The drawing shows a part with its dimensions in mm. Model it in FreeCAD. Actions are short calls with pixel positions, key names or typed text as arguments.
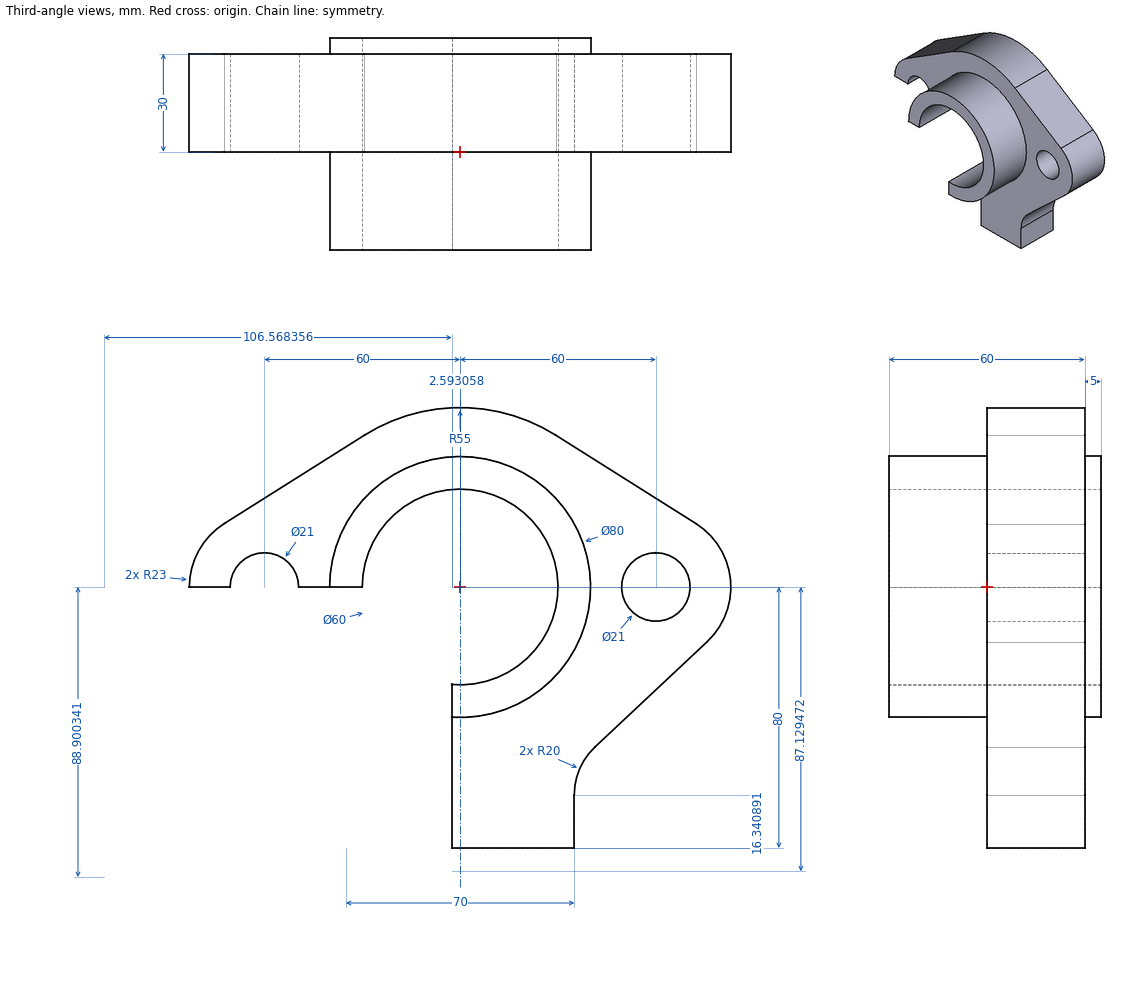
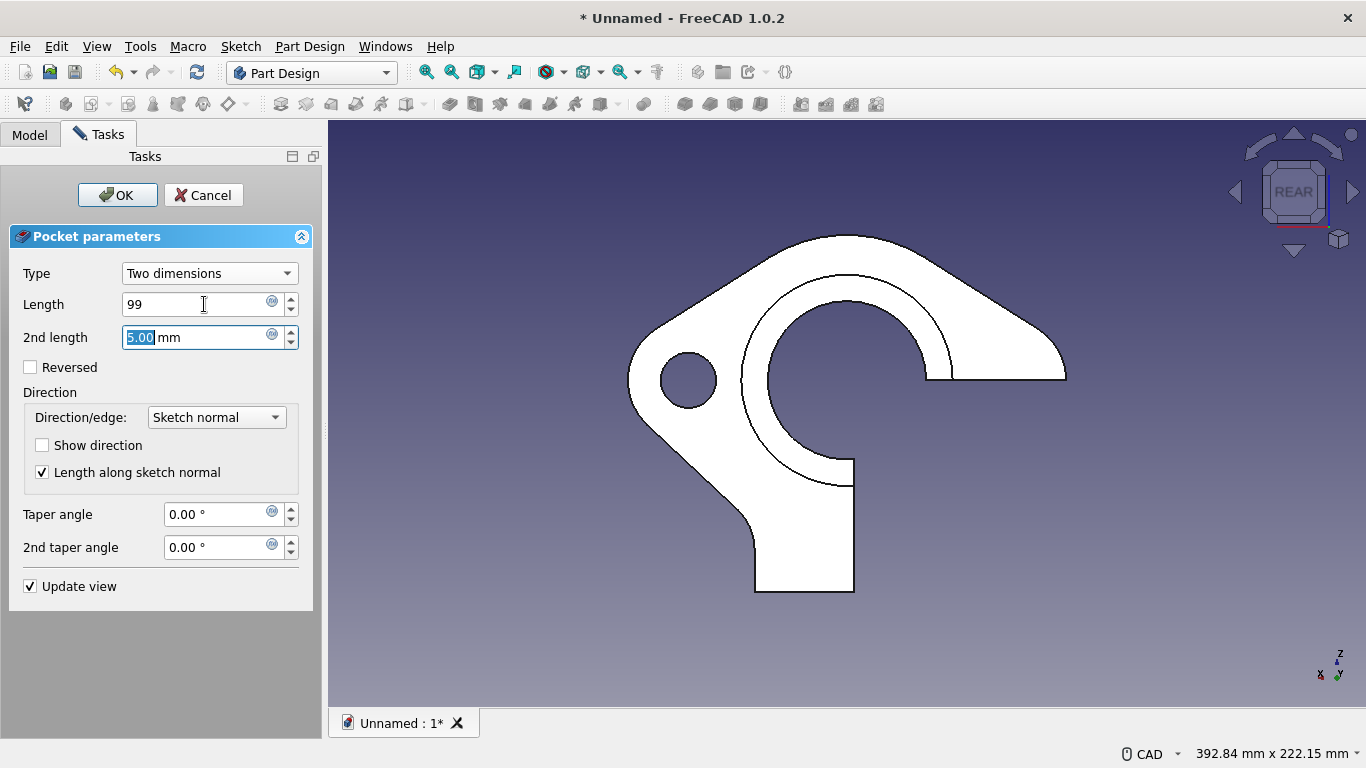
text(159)
key(Tab)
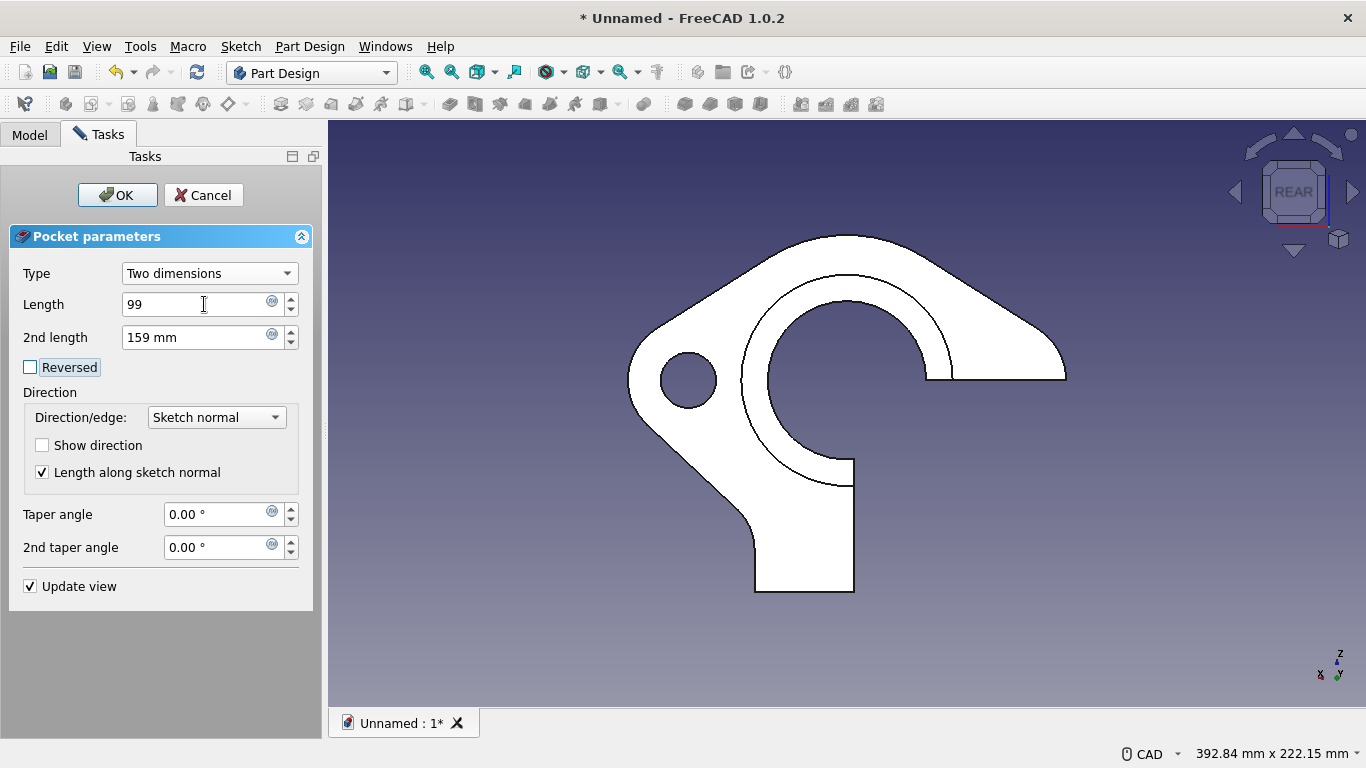
click(31, 367)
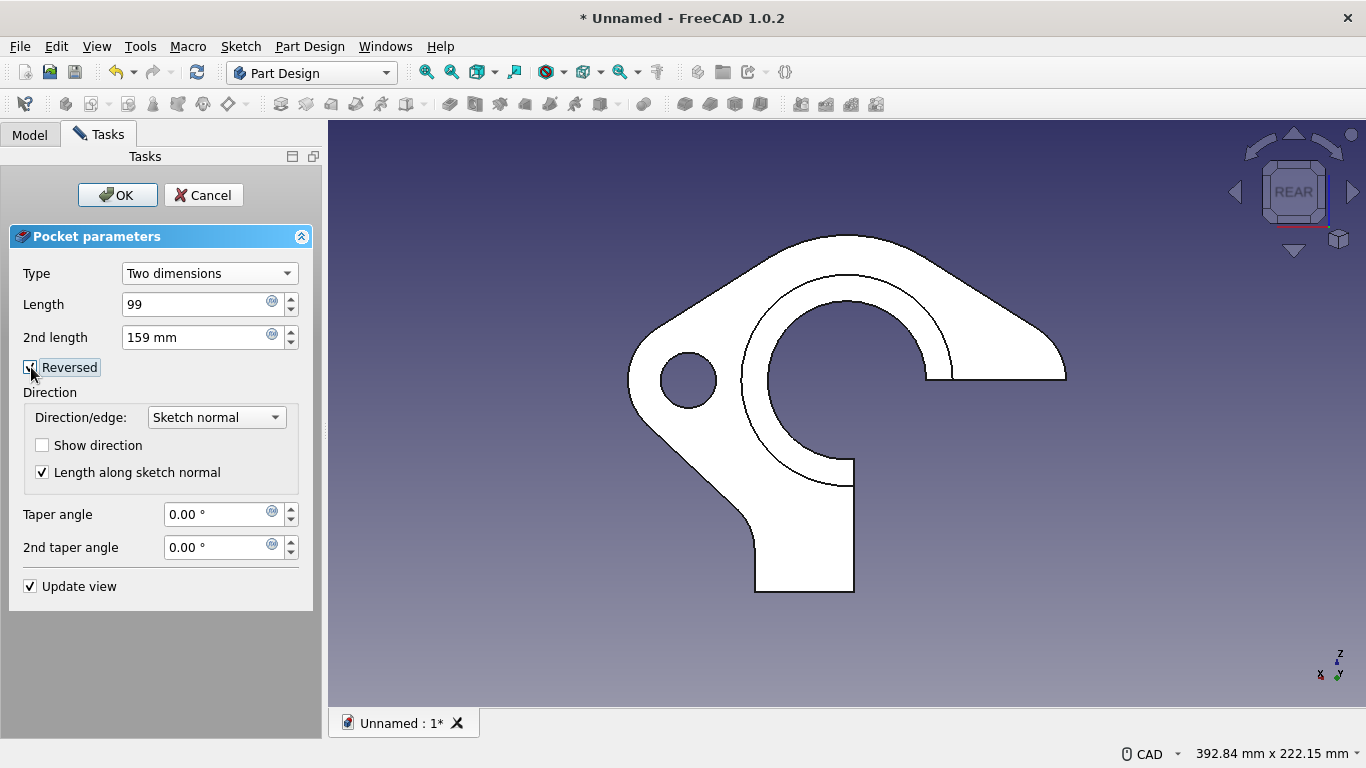
click(118, 195)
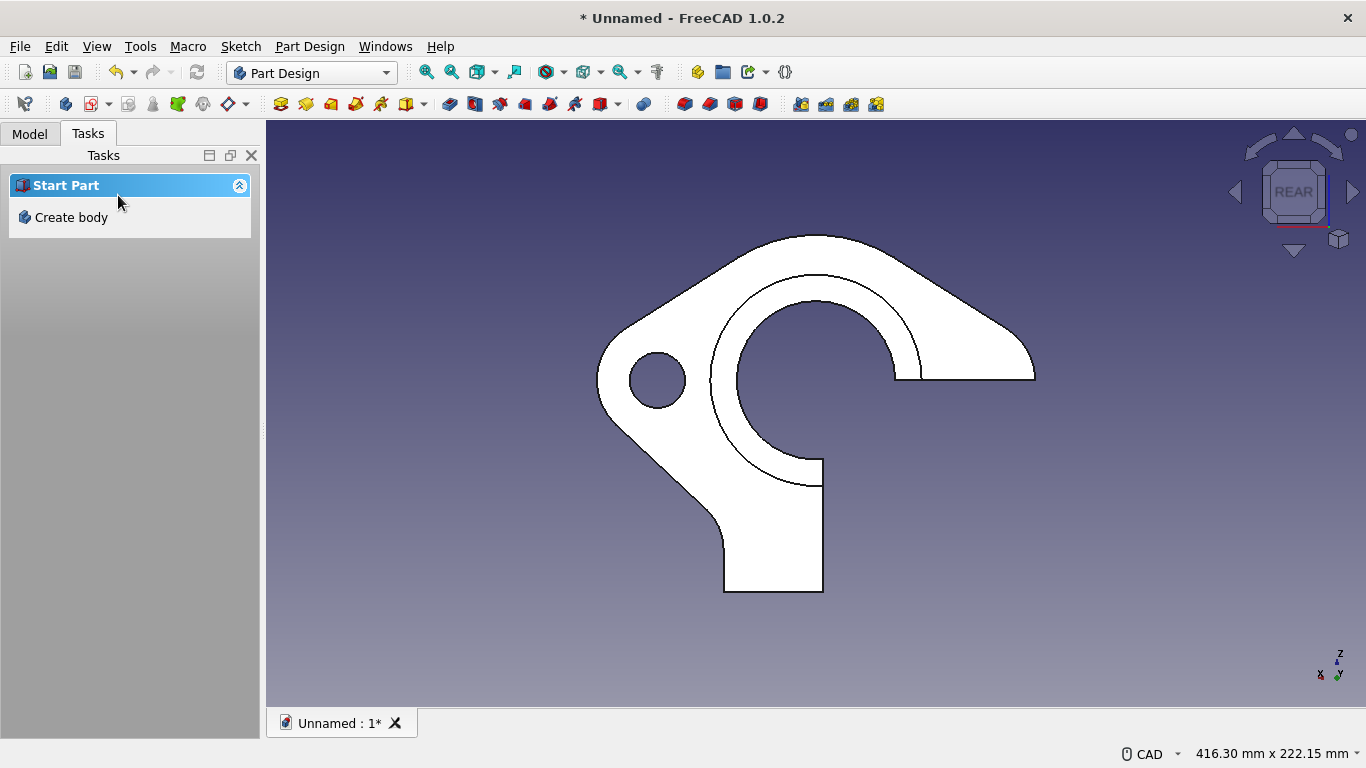
click(90, 104)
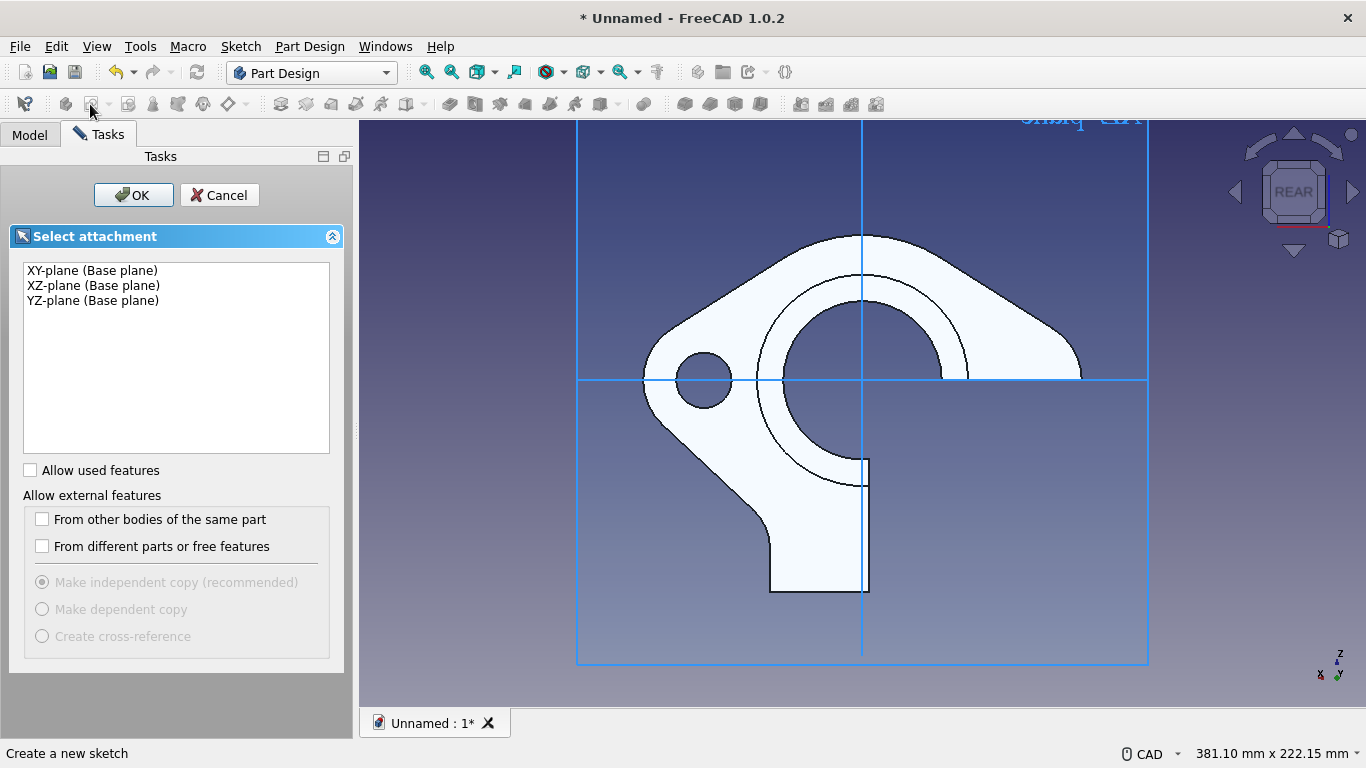
click(84, 286)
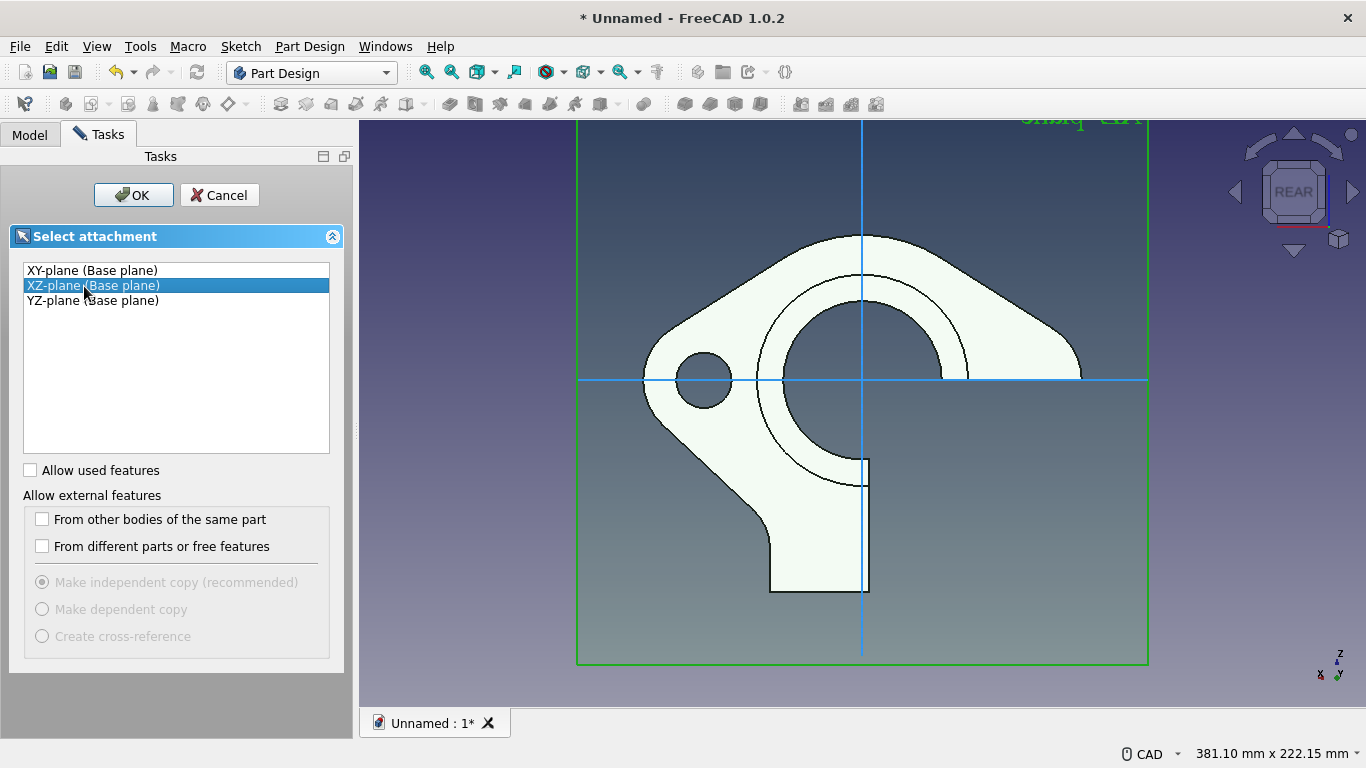
click(134, 195)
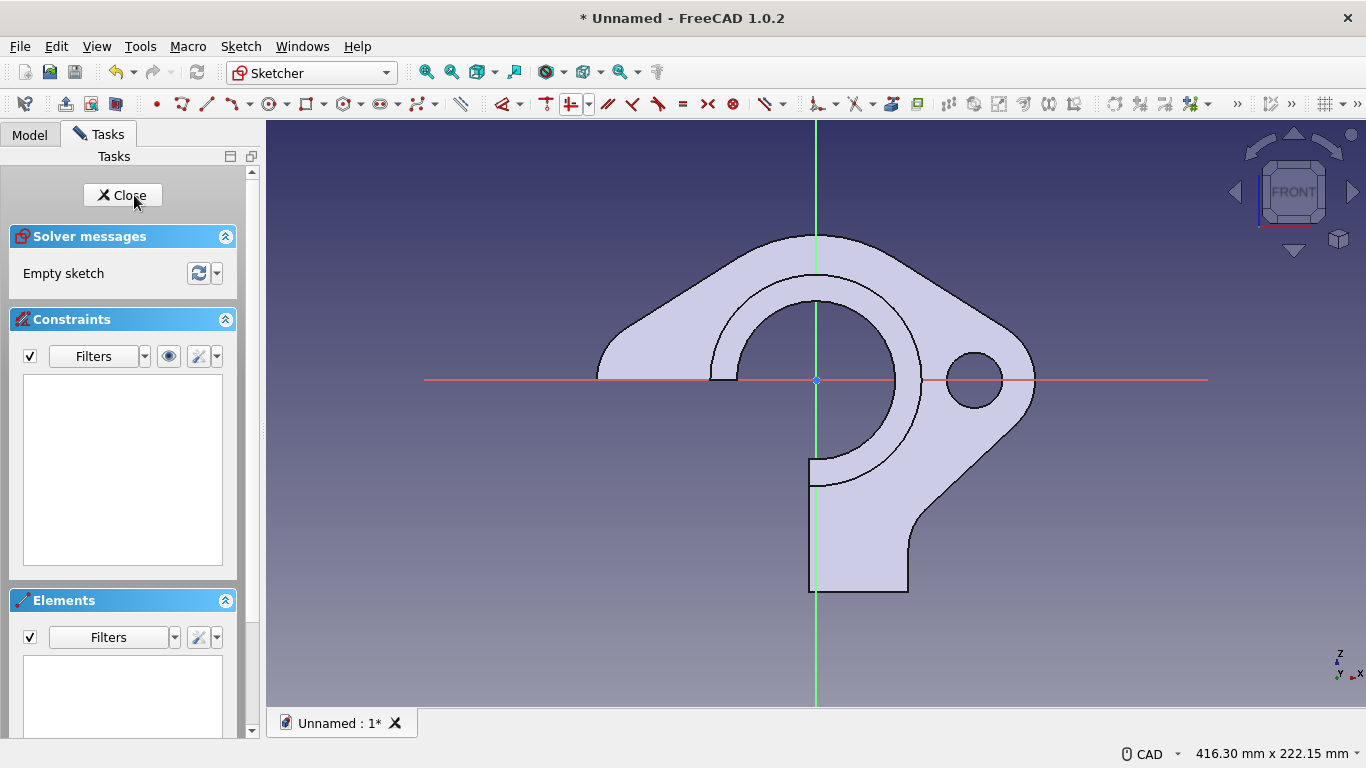
click(116, 104)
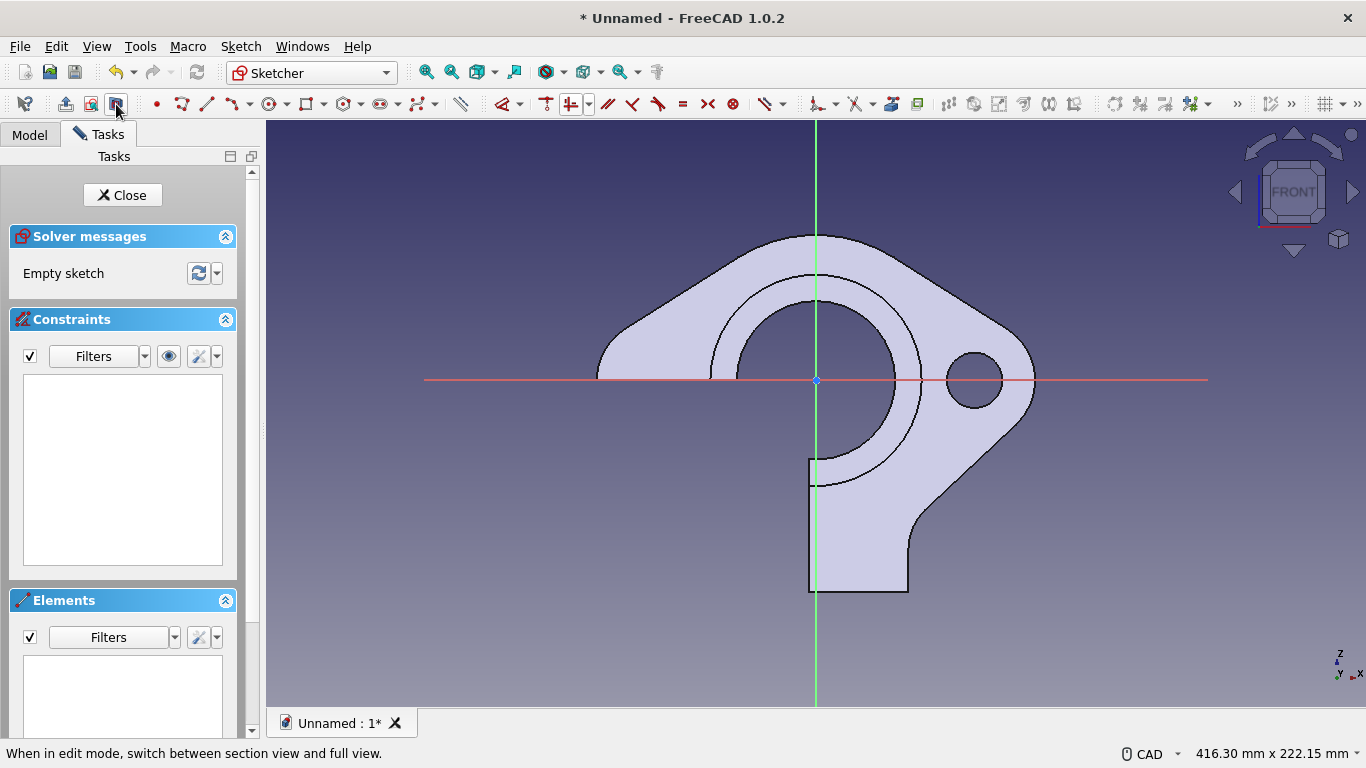
scroll(643, 375, up, 10)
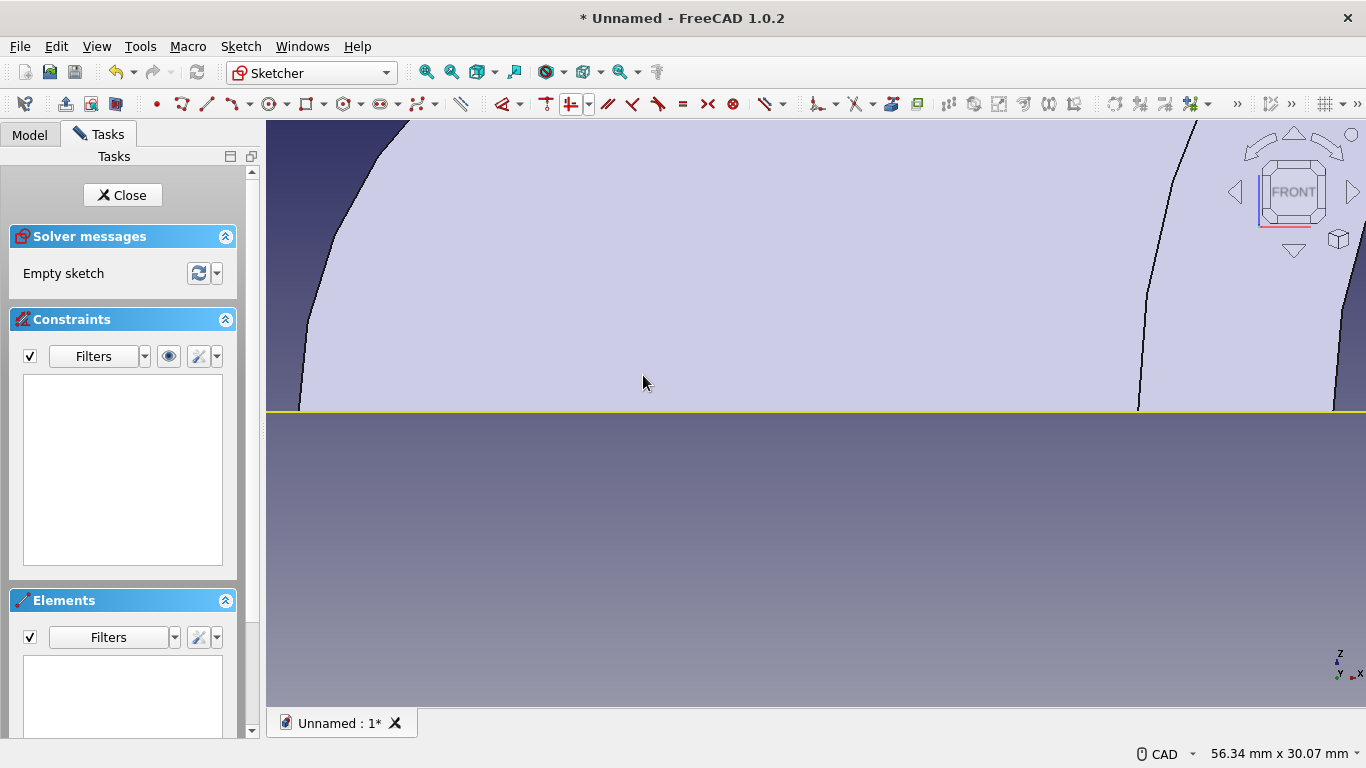
click(268, 104)